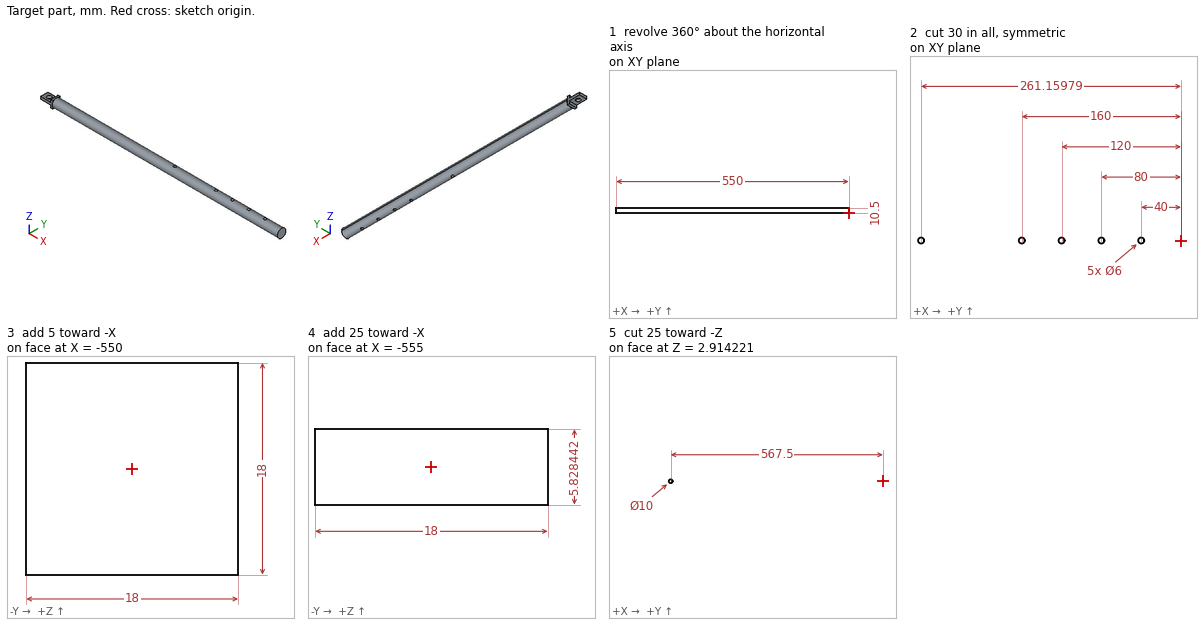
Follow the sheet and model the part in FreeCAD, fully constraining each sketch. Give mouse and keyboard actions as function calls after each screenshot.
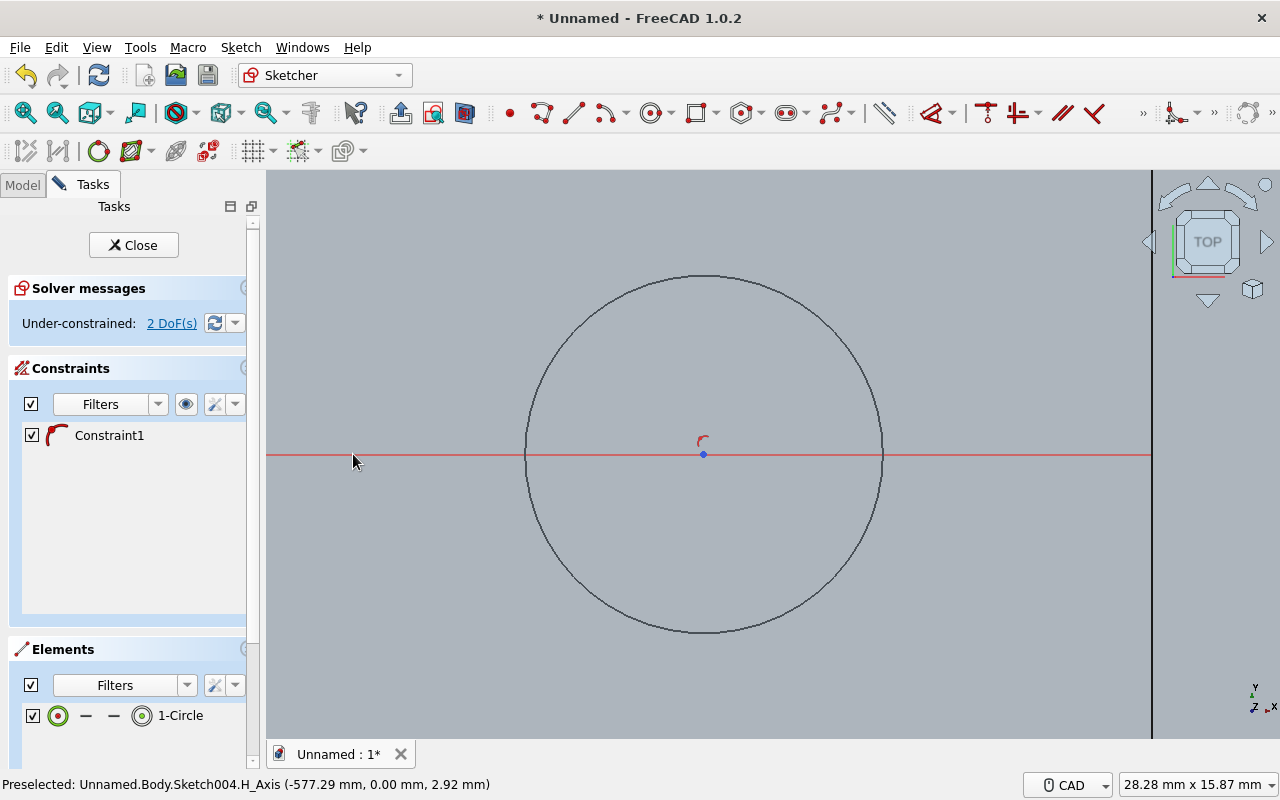
key(d)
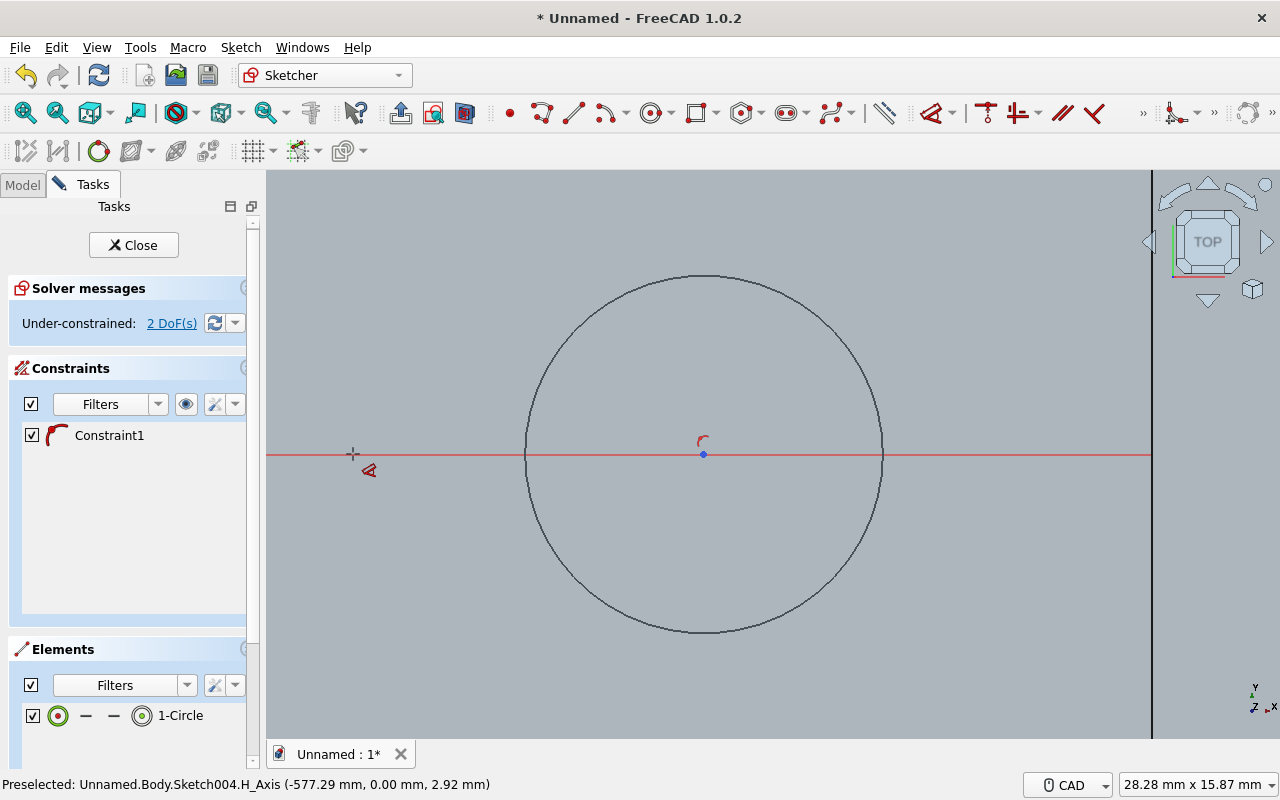
click(830, 328)
click(853, 305)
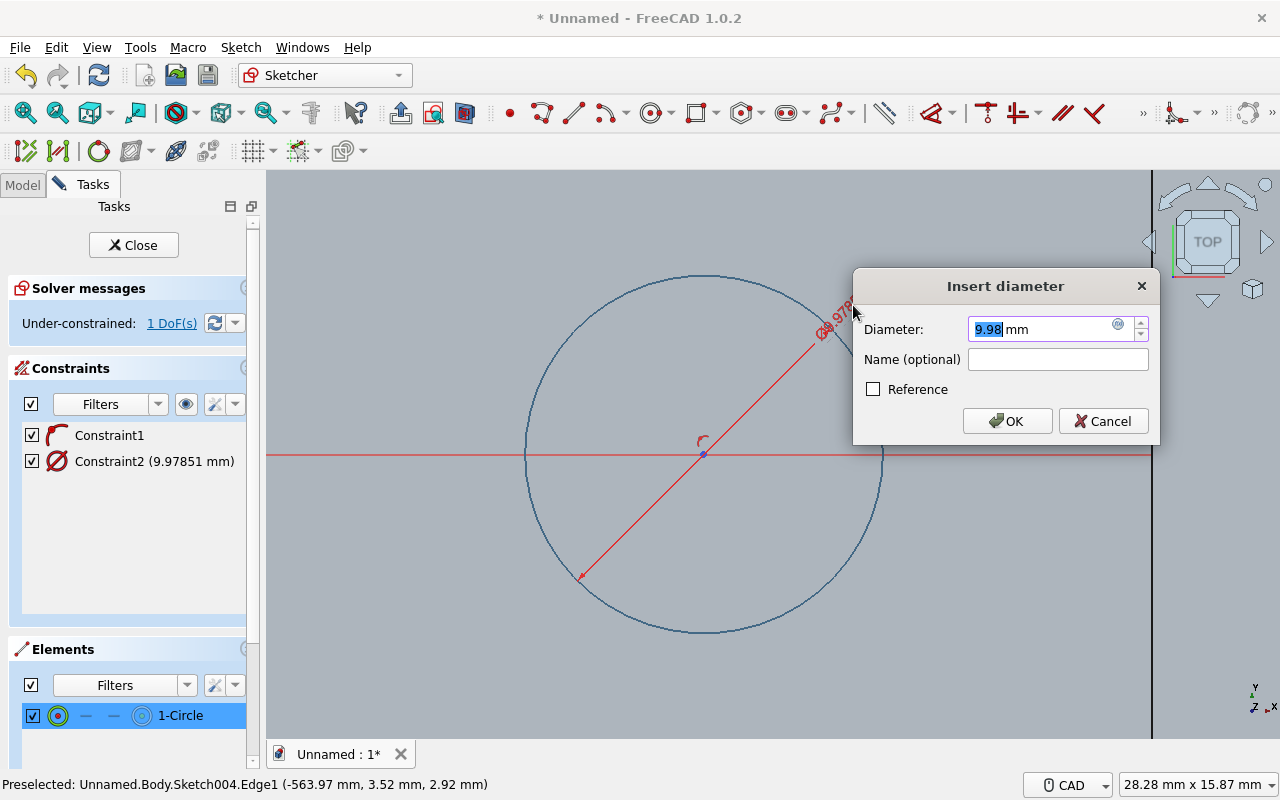
text(10)
key(Return)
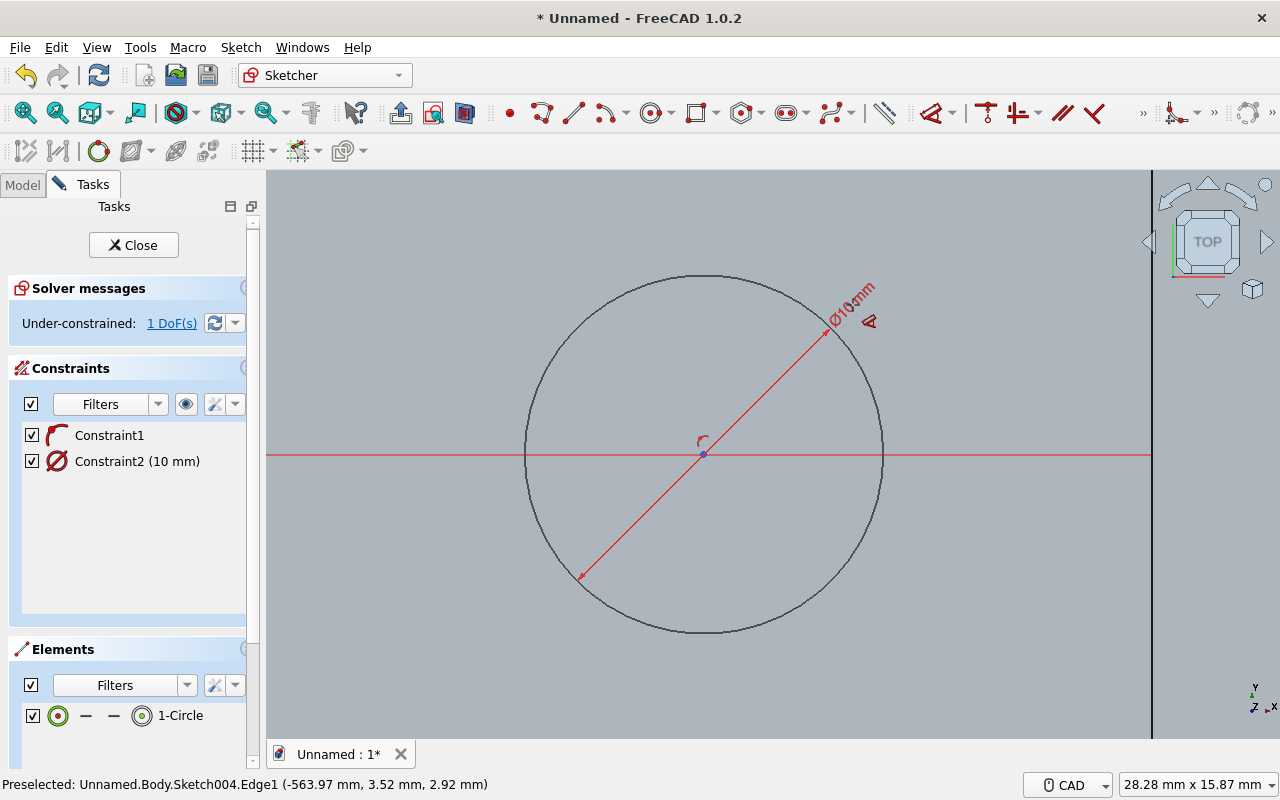
click(704, 454)
click(909, 488)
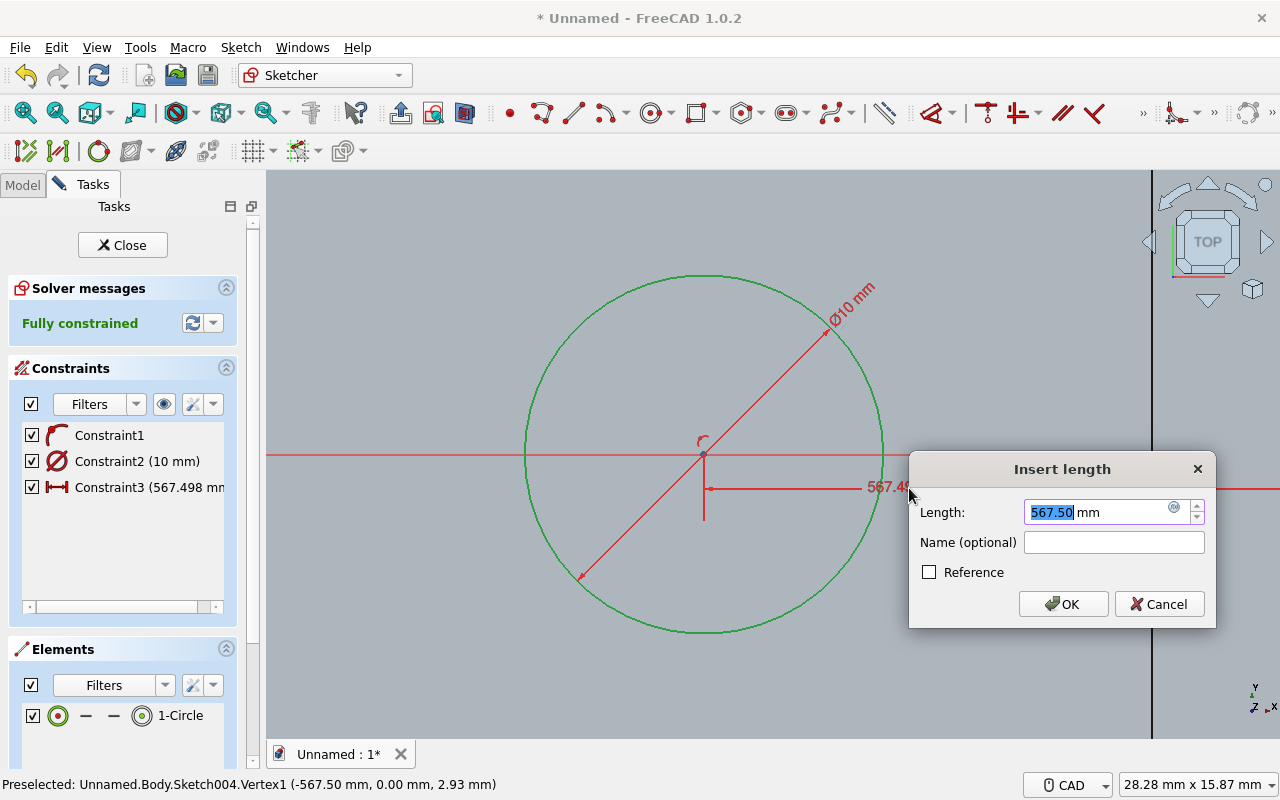
text(567.5)
key(Return)
key(Escape)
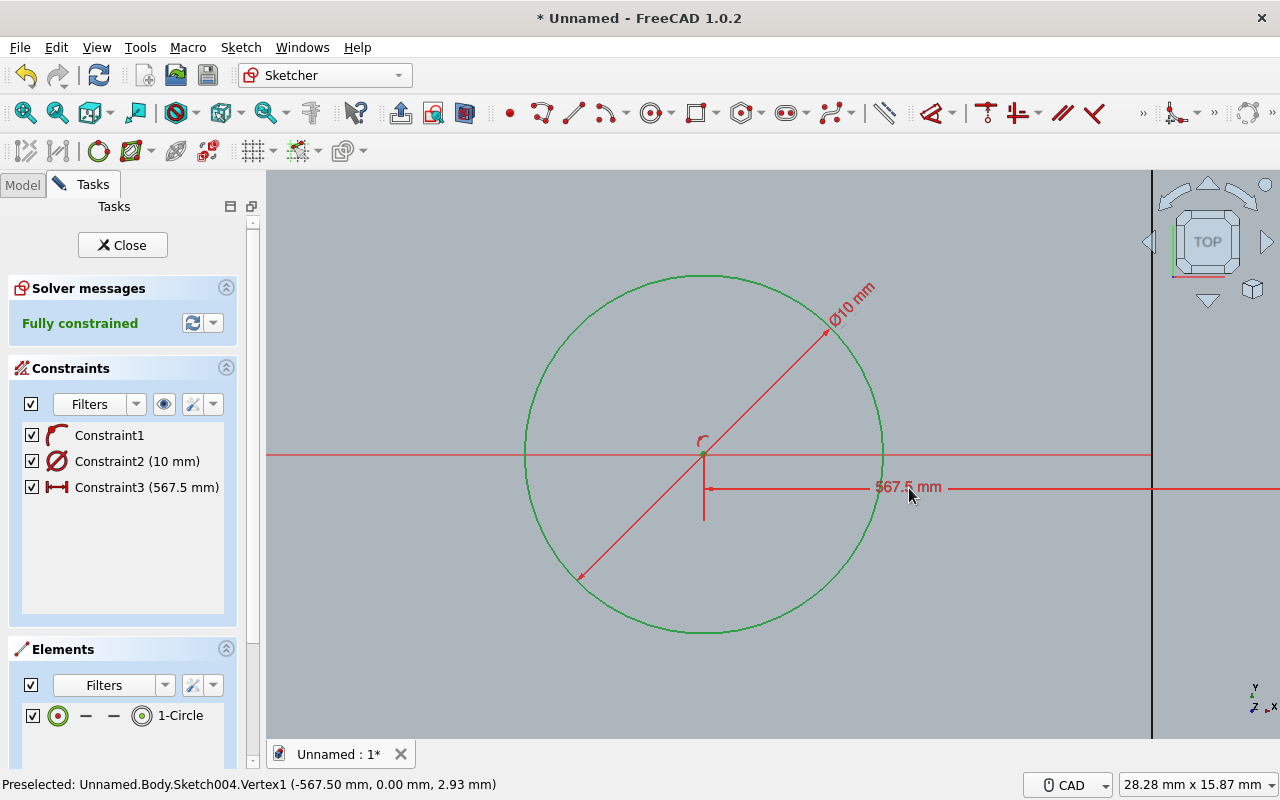
click(123, 245)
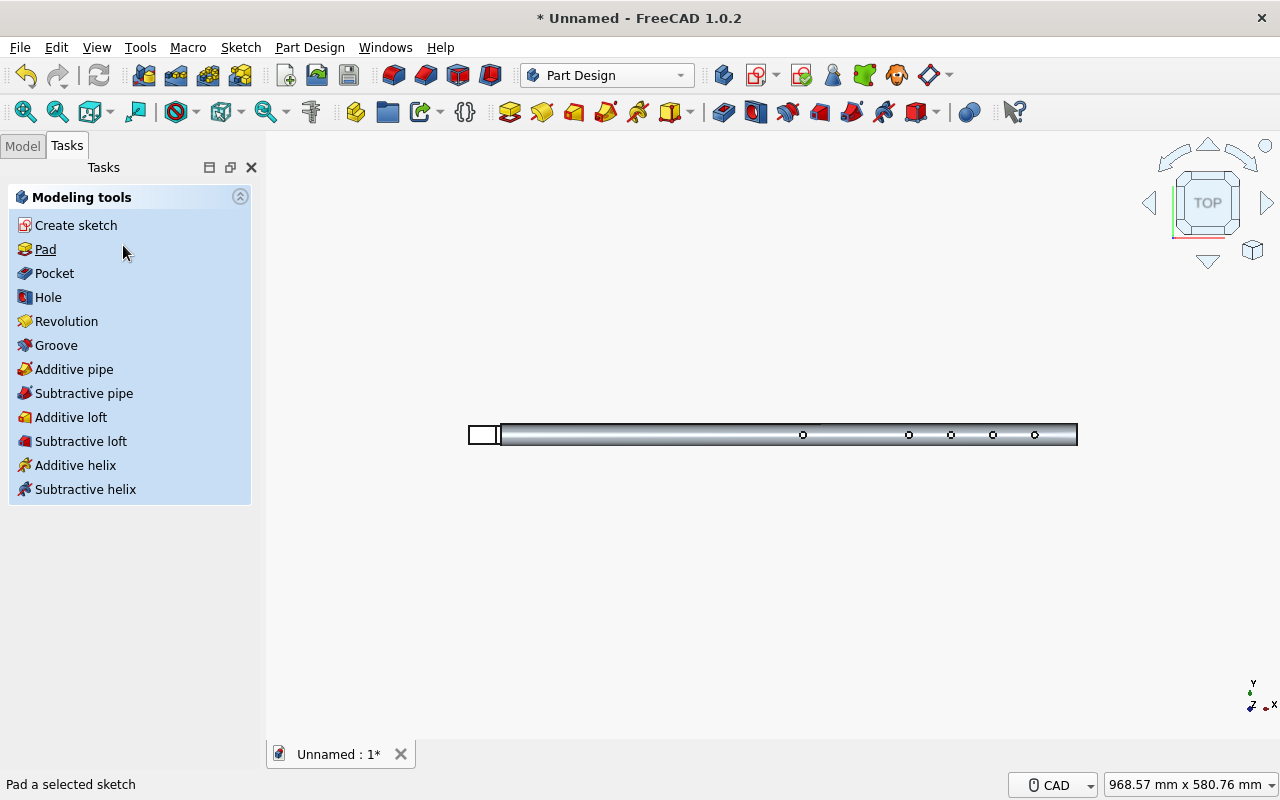
click(724, 112)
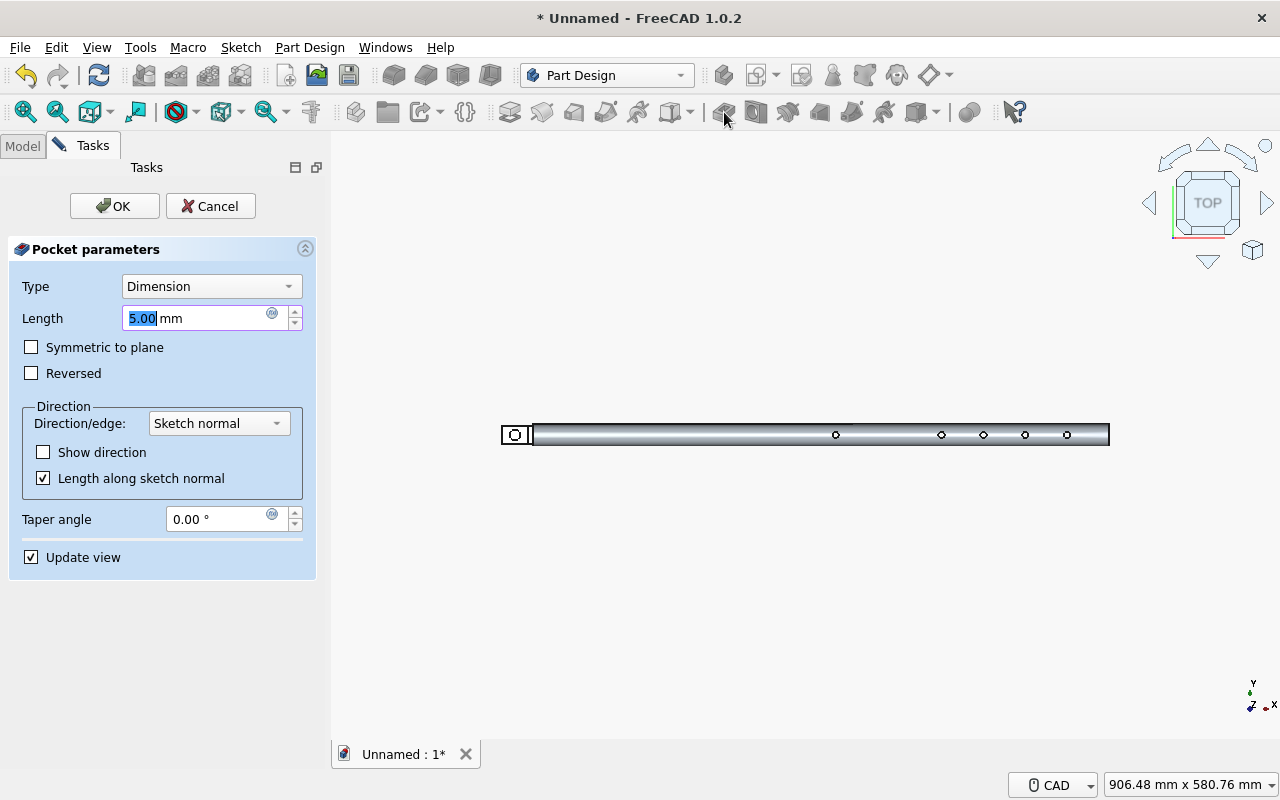
text(25)
key(Tab)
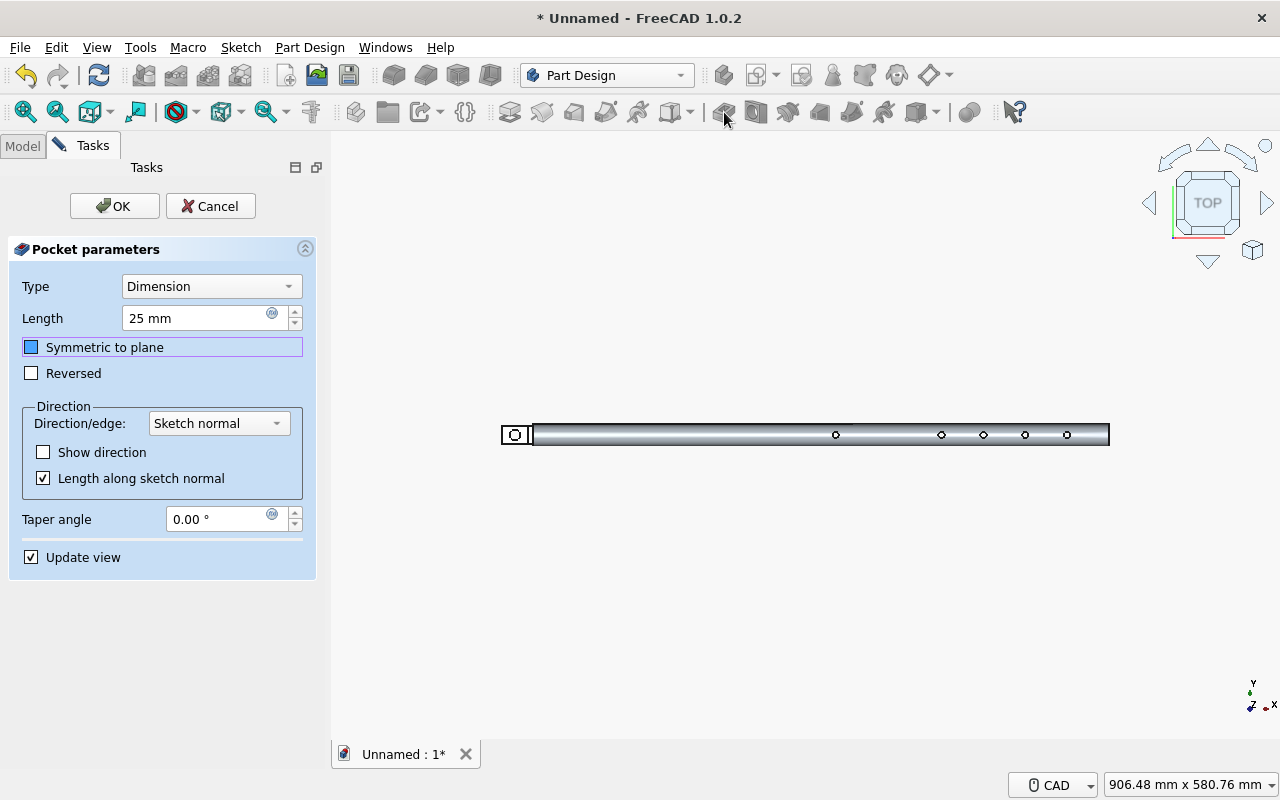
click(115, 206)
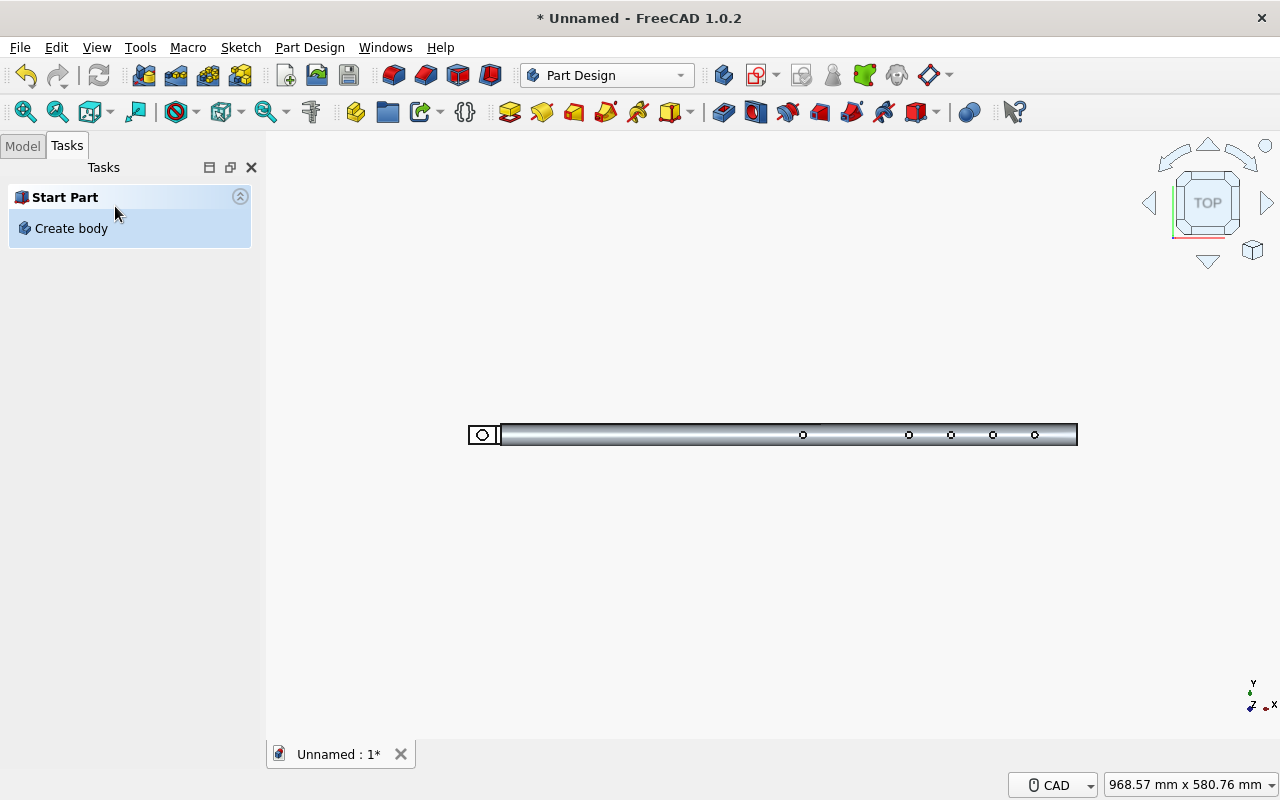
key(0)